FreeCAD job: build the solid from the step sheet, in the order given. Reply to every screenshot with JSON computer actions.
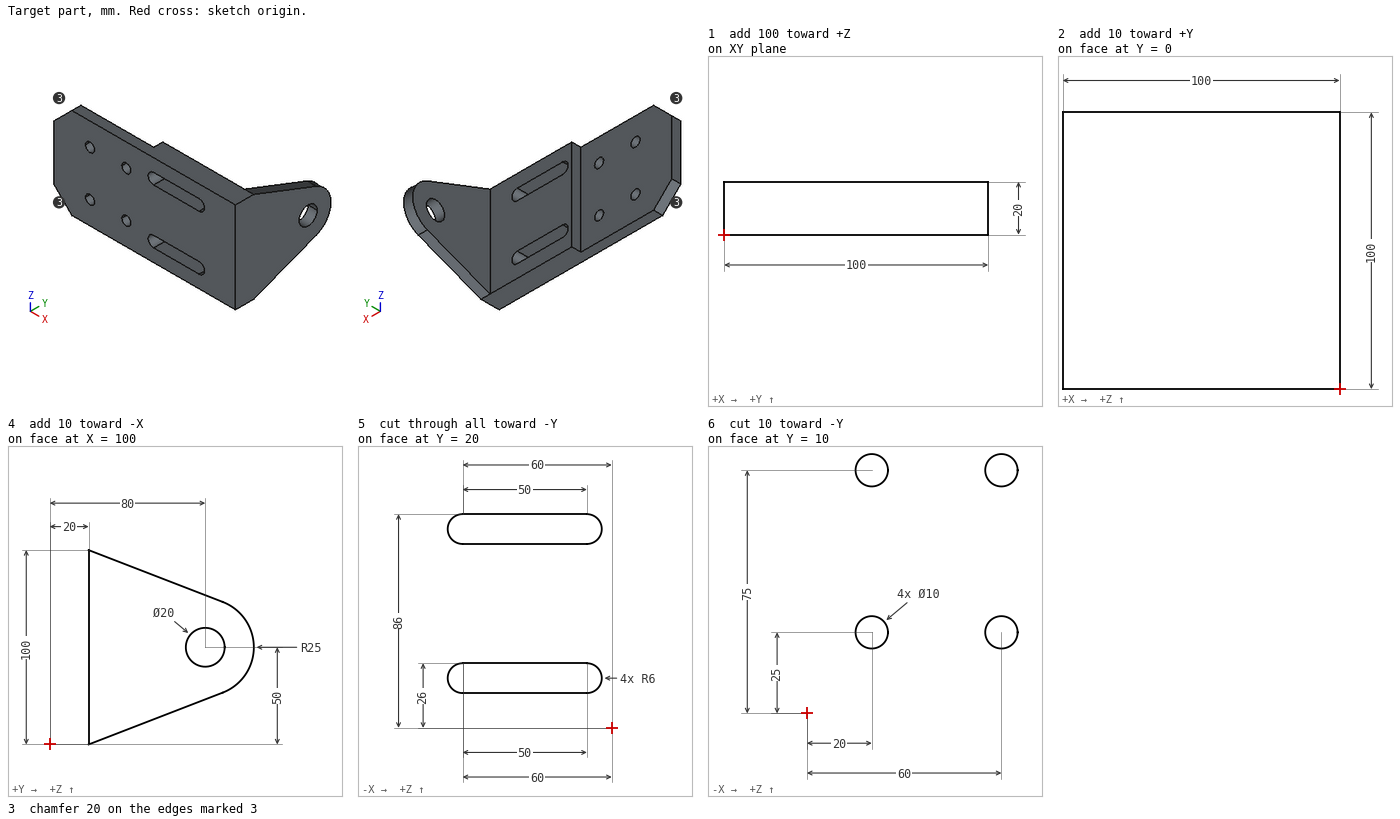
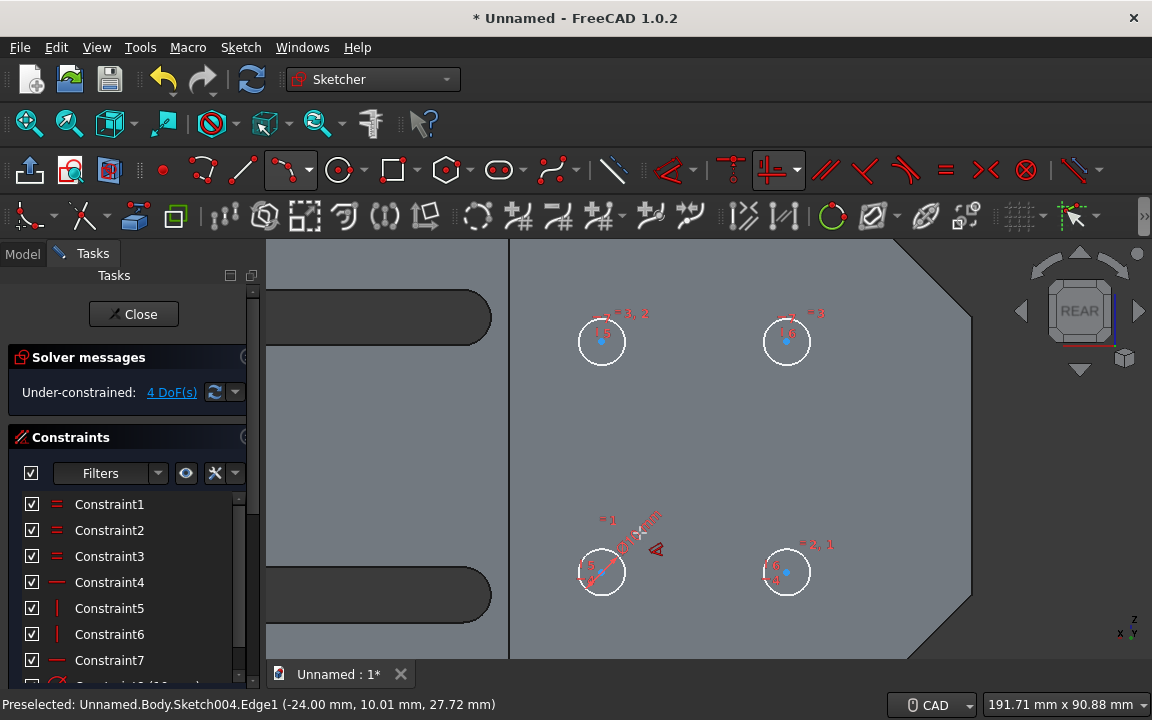
{"action": "left_click", "coordinate": [602, 572]}
{"action": "left_click", "coordinate": [556, 538]}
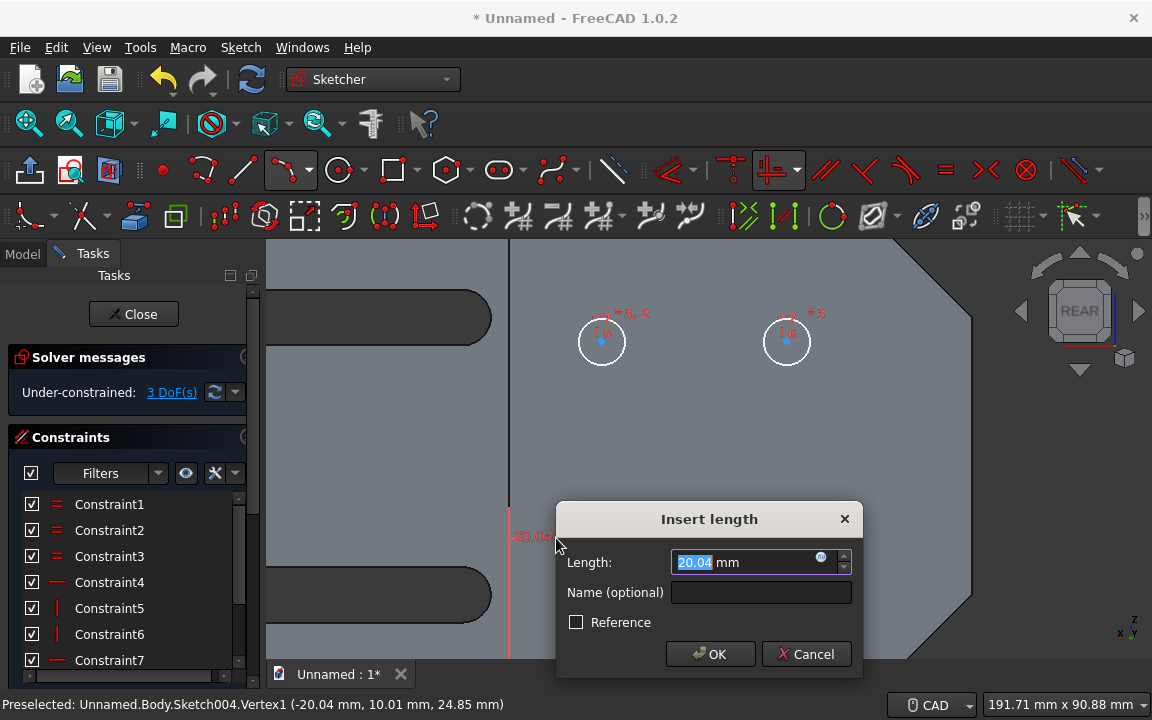
{"action": "type", "text": "20"}
{"action": "key", "text": "Return"}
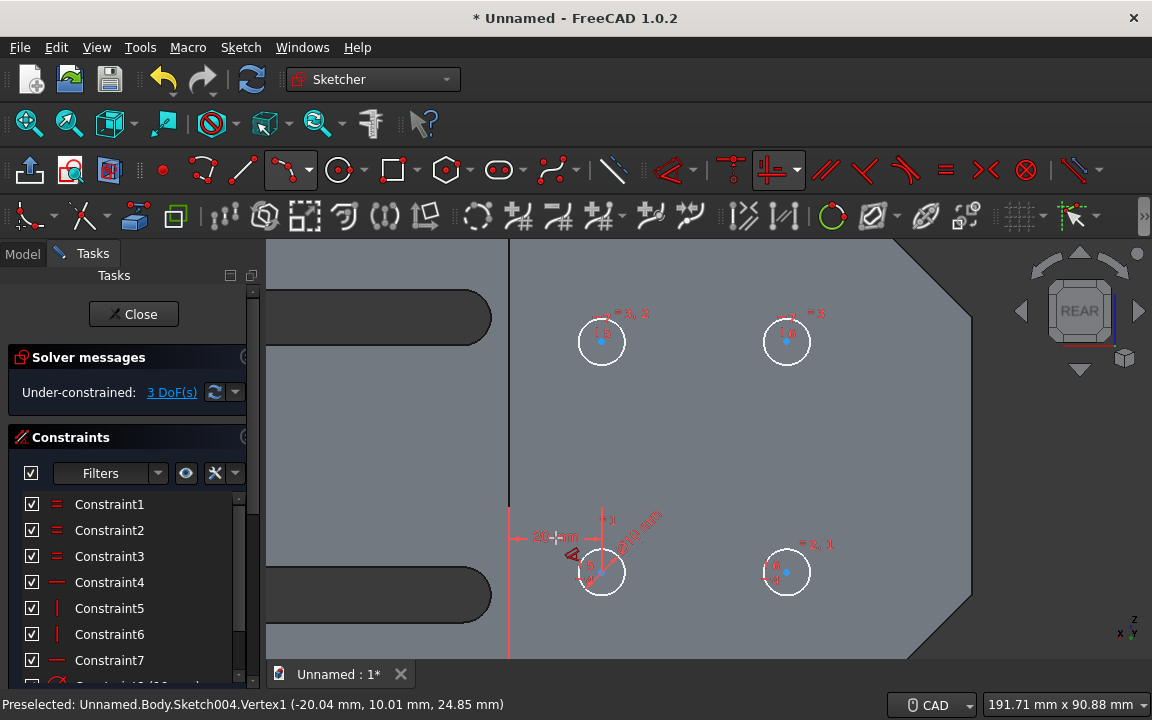
{"action": "left_click", "coordinate": [602, 572]}
{"action": "left_click", "coordinate": [475, 602]}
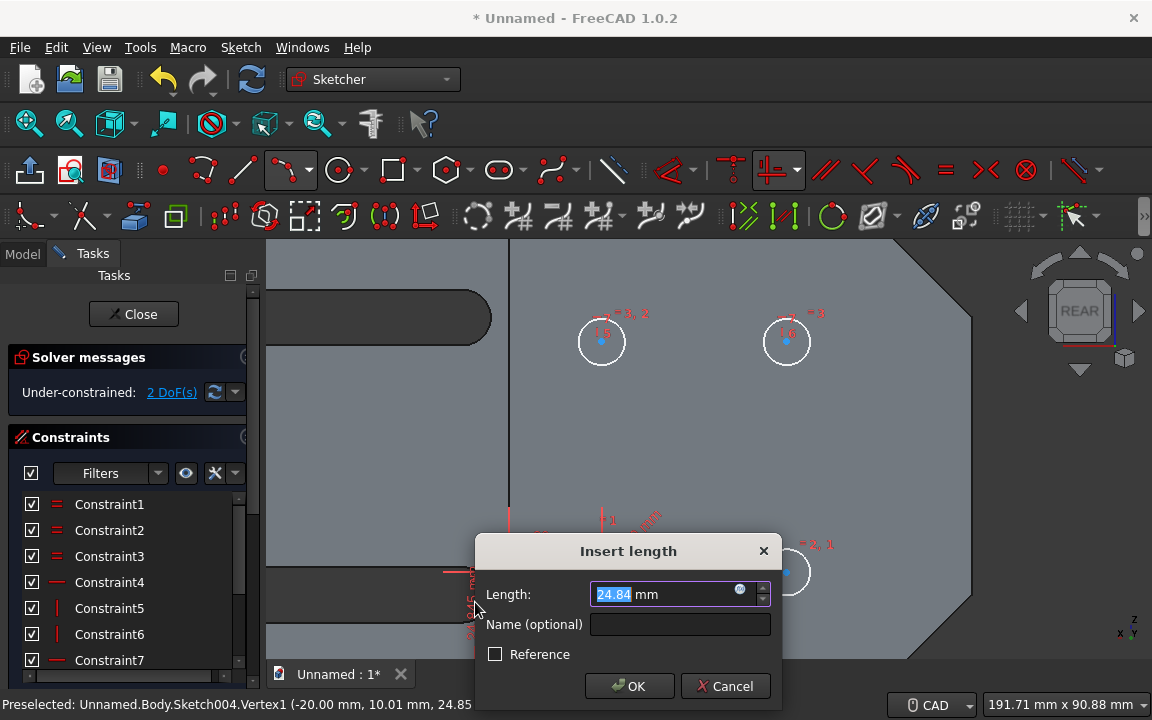
{"action": "type", "text": "25"}
{"action": "key", "text": "Return"}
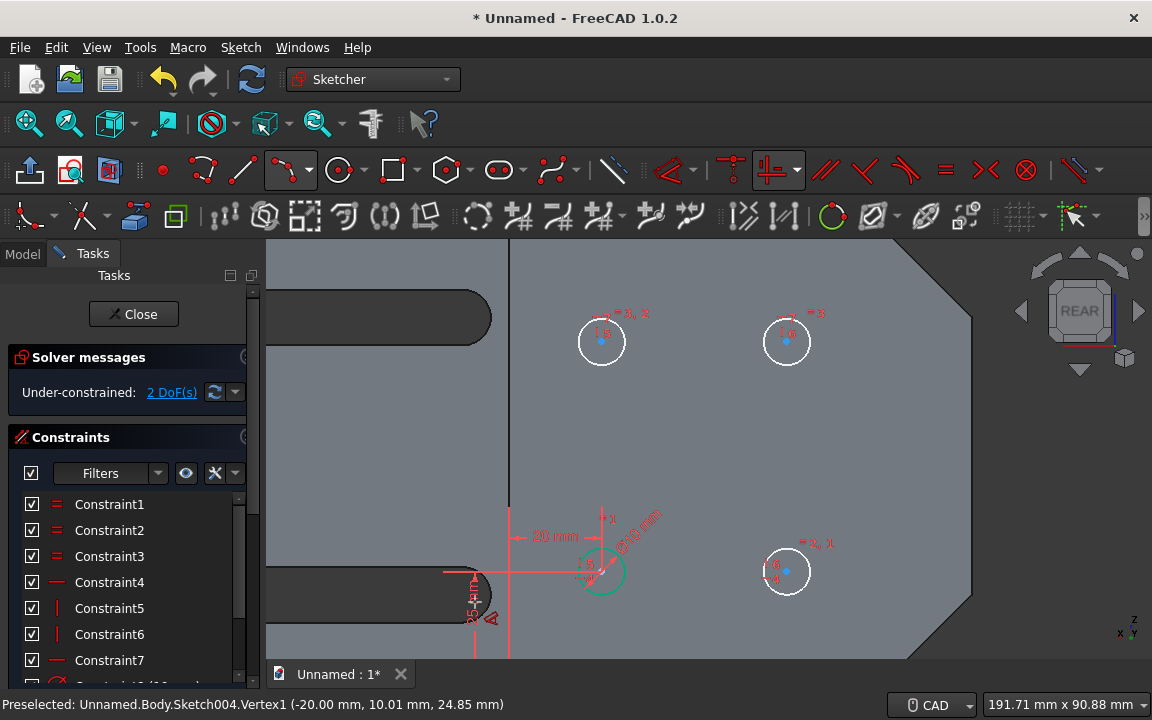
{"action": "left_click", "coordinate": [787, 572]}
{"action": "left_click", "coordinate": [712, 538]}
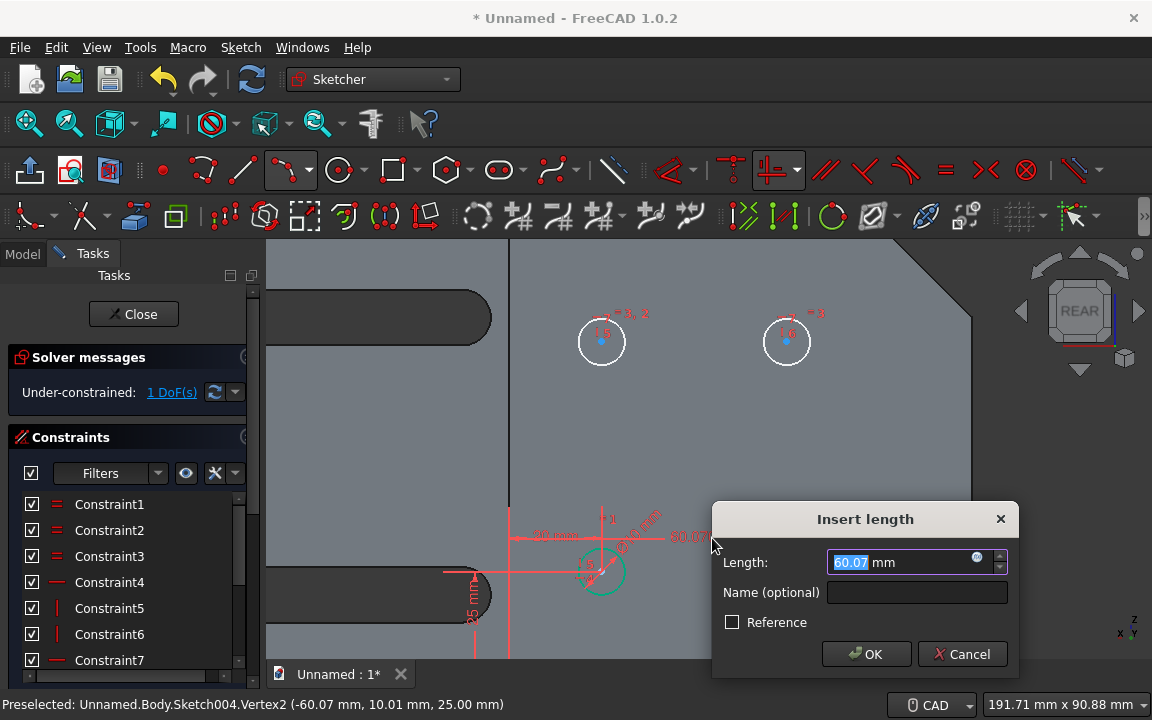
{"action": "type", "text": "60"}
{"action": "key", "text": "Return"}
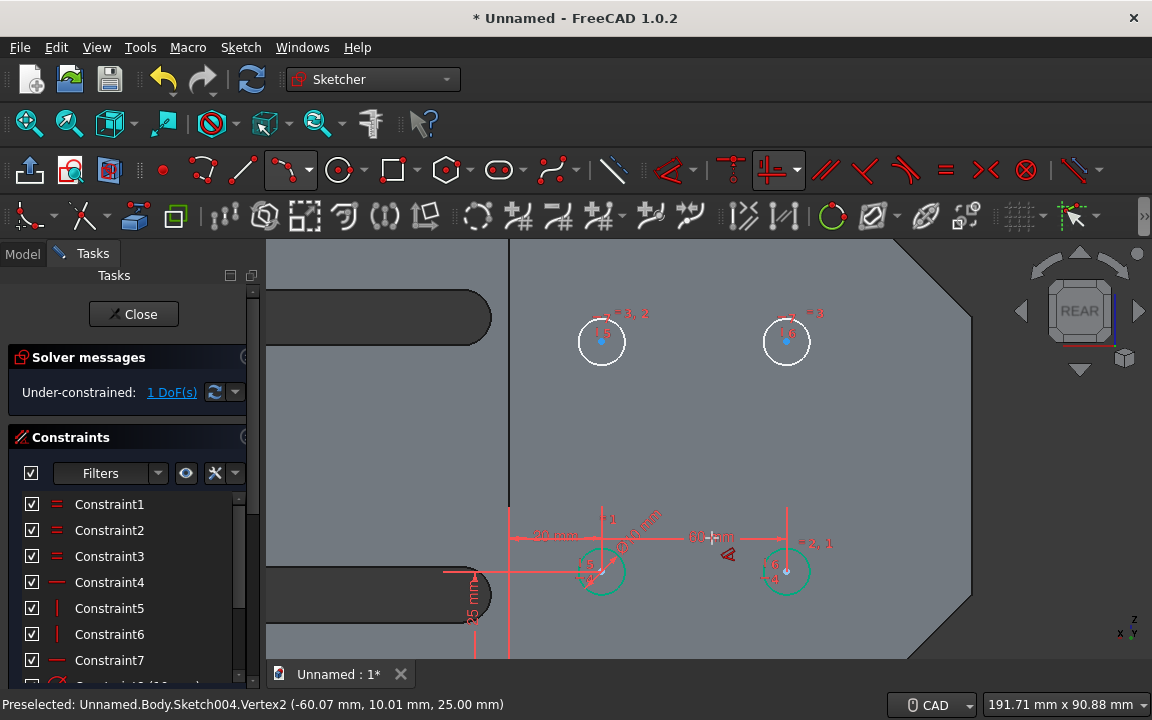
{"action": "left_click", "coordinate": [602, 342]}
{"action": "left_click", "coordinate": [475, 487]}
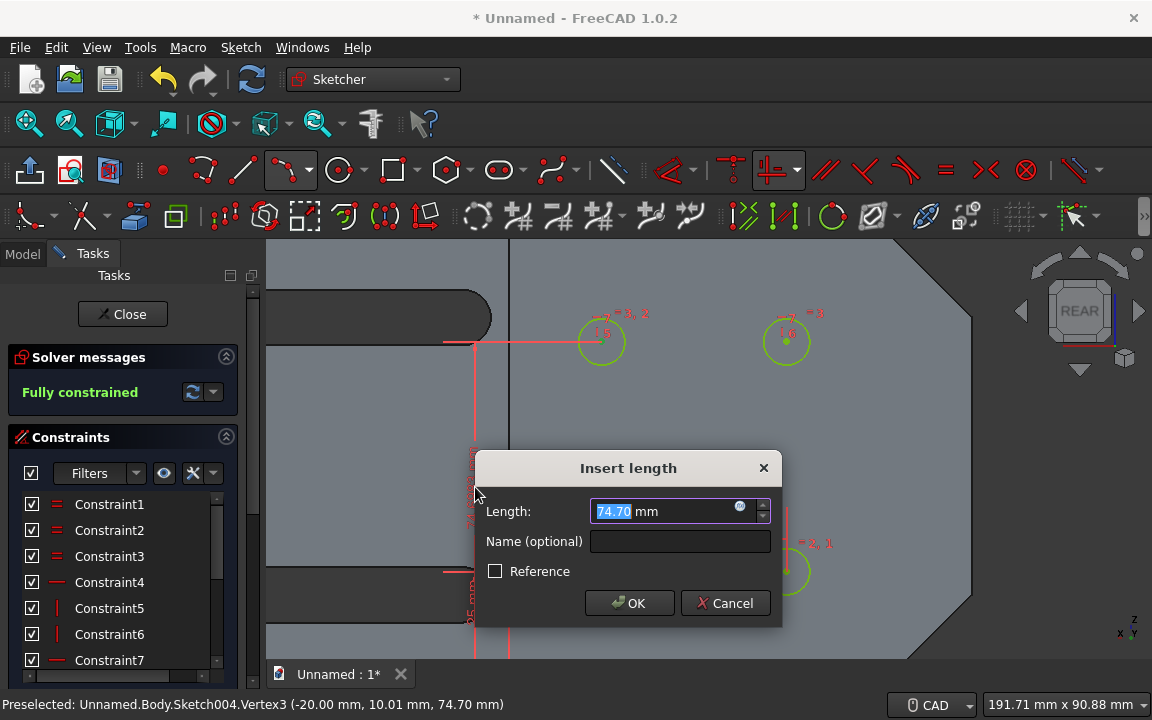
{"action": "type", "text": "75"}
{"action": "key", "text": "Return"}
{"action": "key", "text": "Escape"}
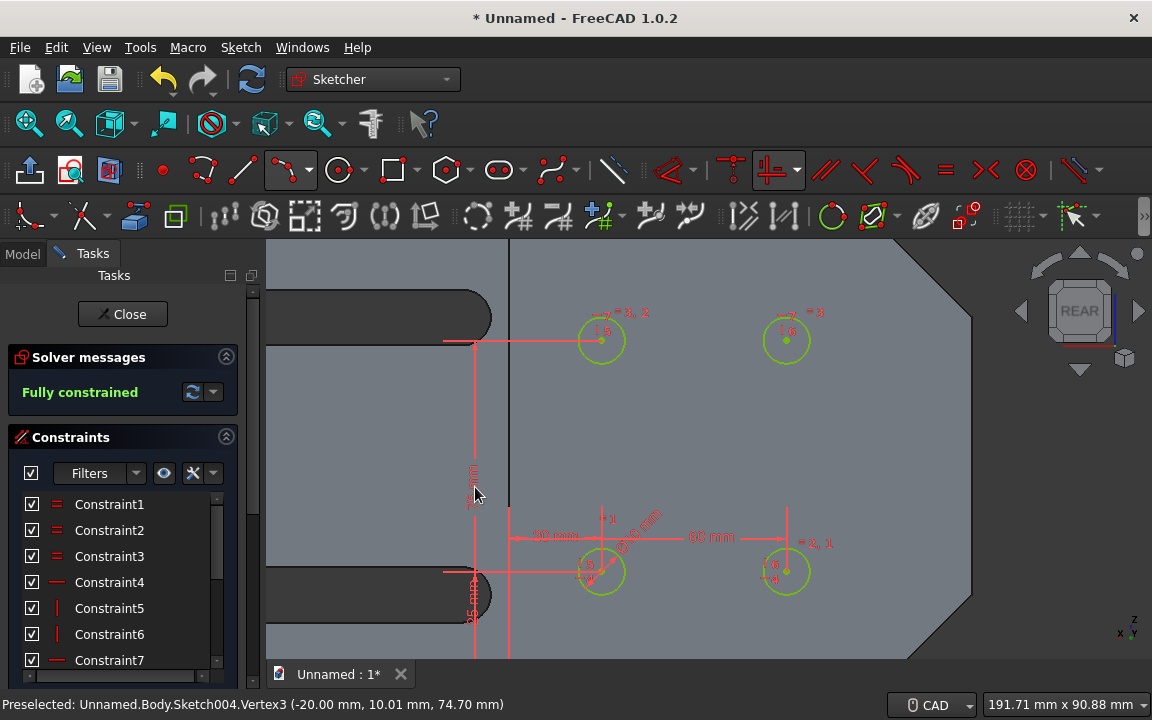
{"action": "left_click", "coordinate": [123, 314]}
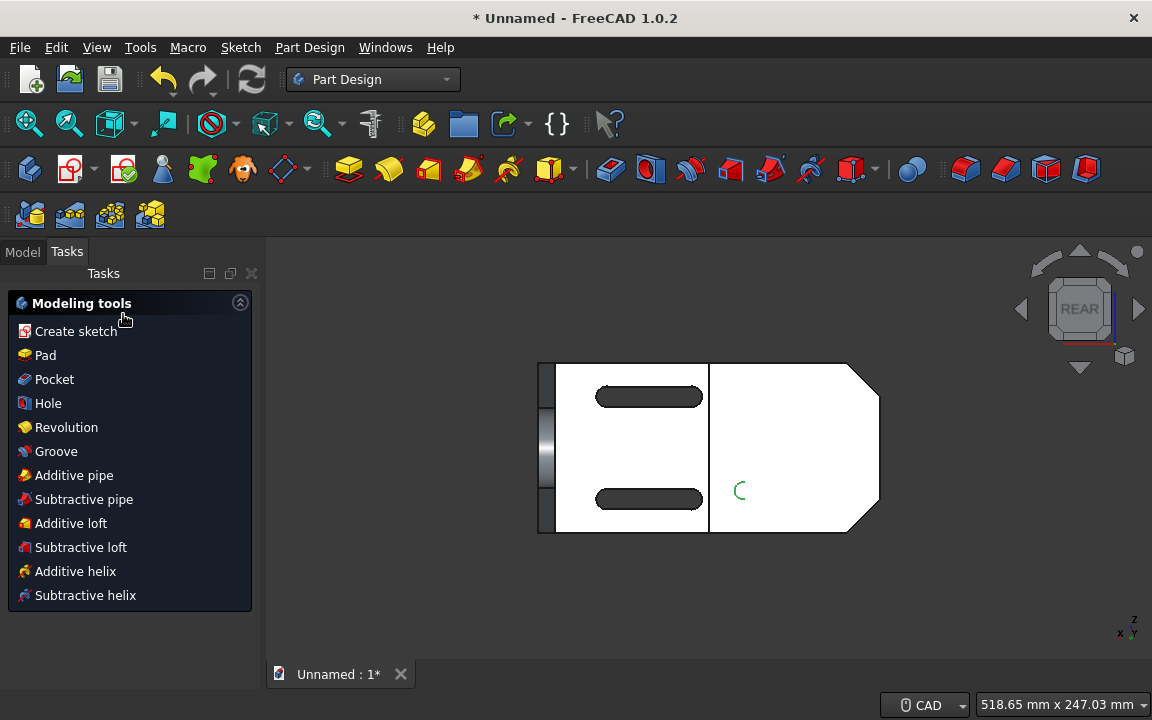
{"action": "left_click", "coordinate": [612, 170]}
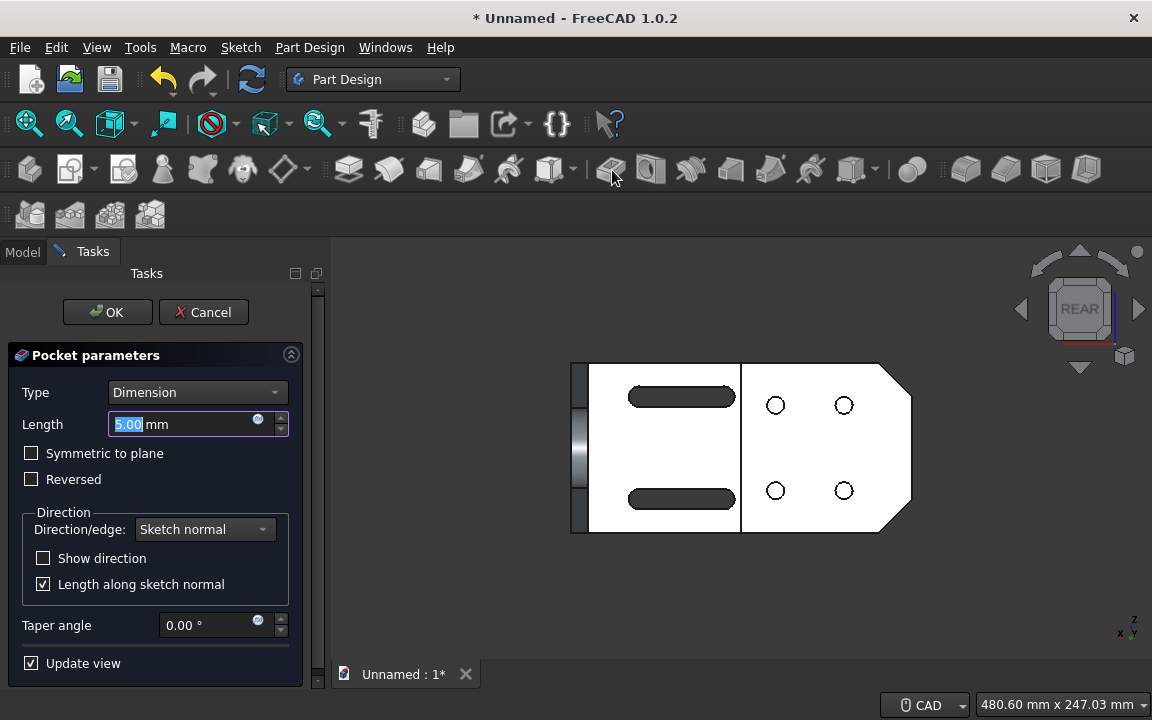
{"action": "type", "text": "10"}
{"action": "key", "text": "Tab"}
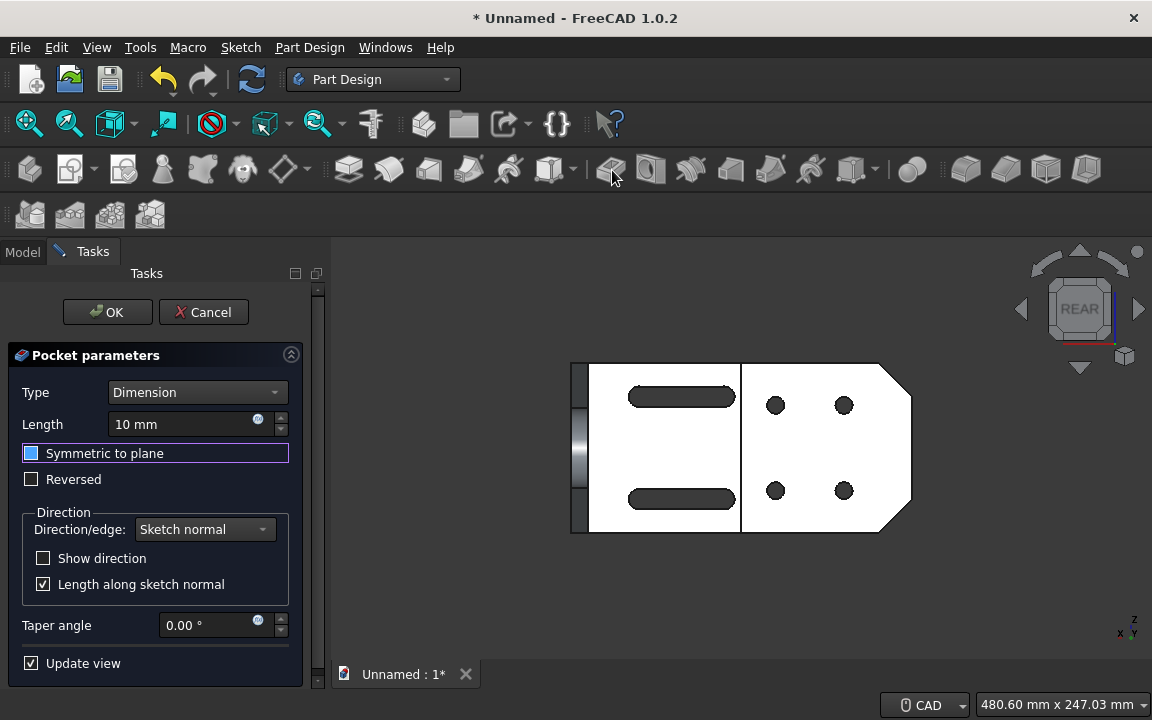
{"action": "left_click", "coordinate": [108, 312]}